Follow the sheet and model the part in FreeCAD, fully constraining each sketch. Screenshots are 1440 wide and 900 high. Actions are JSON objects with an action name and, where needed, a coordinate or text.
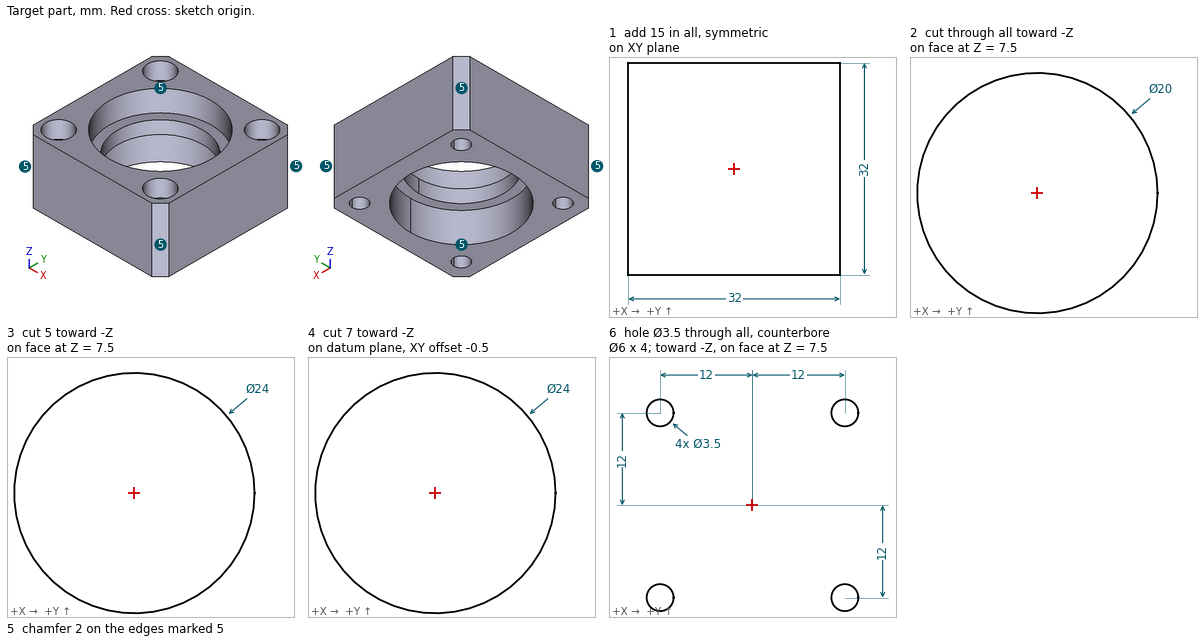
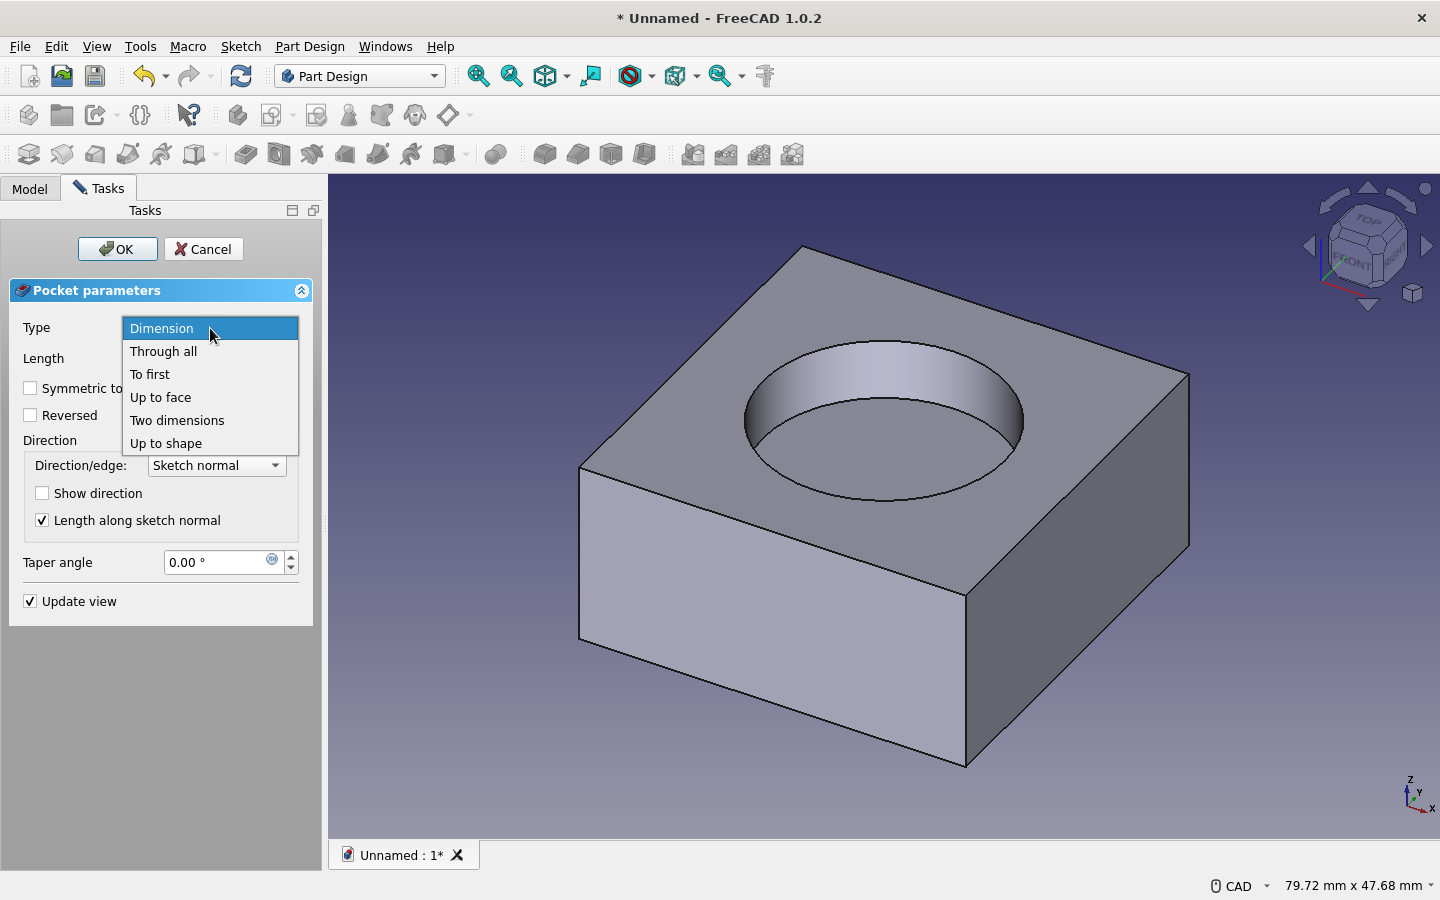
{"action": "left_click", "coordinate": [208, 352]}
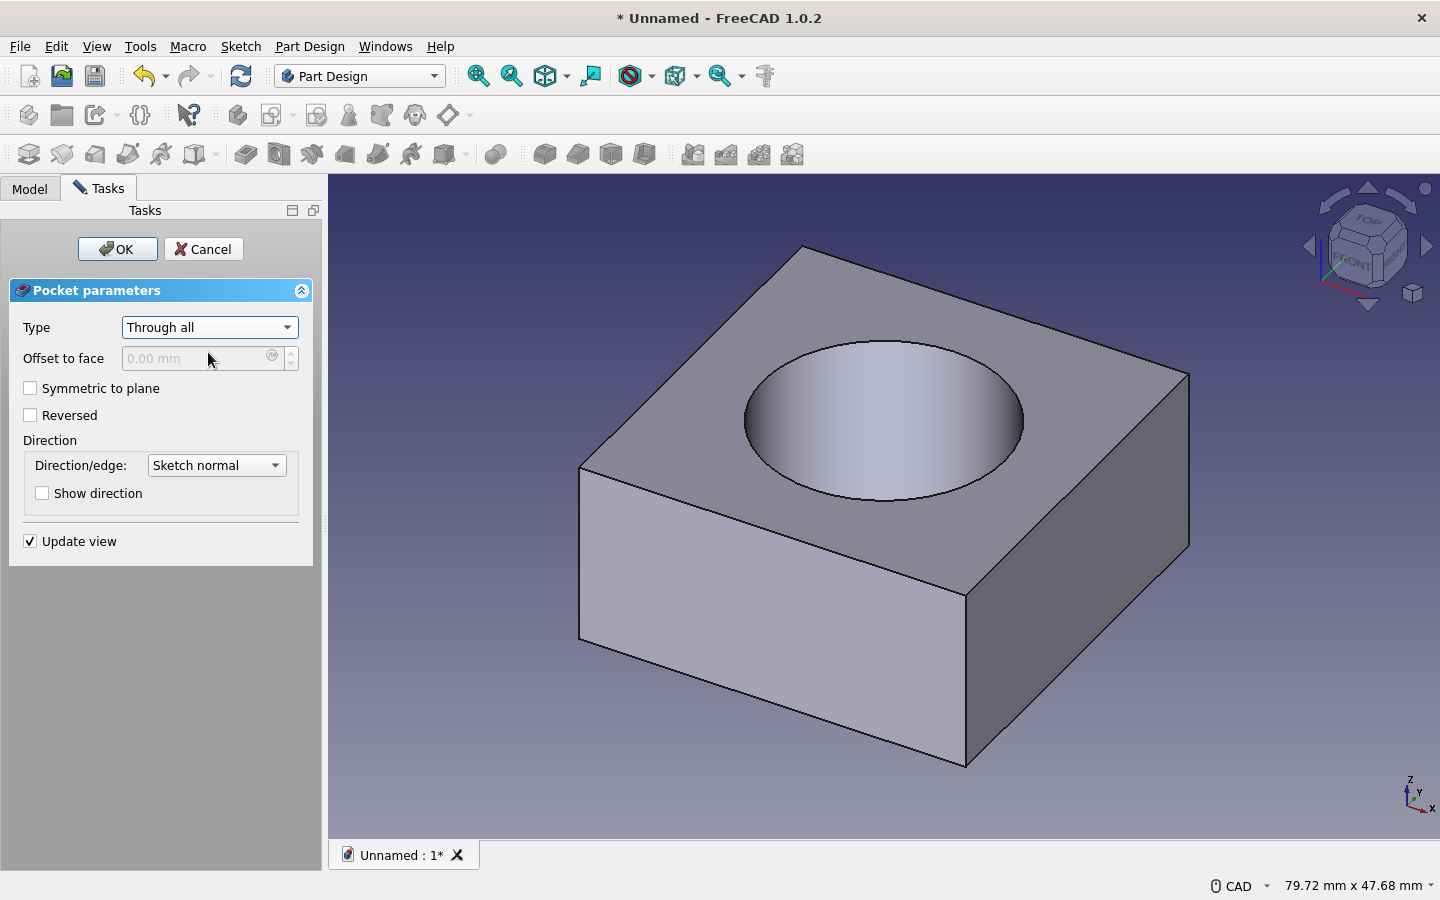
{"action": "left_click", "coordinate": [118, 249]}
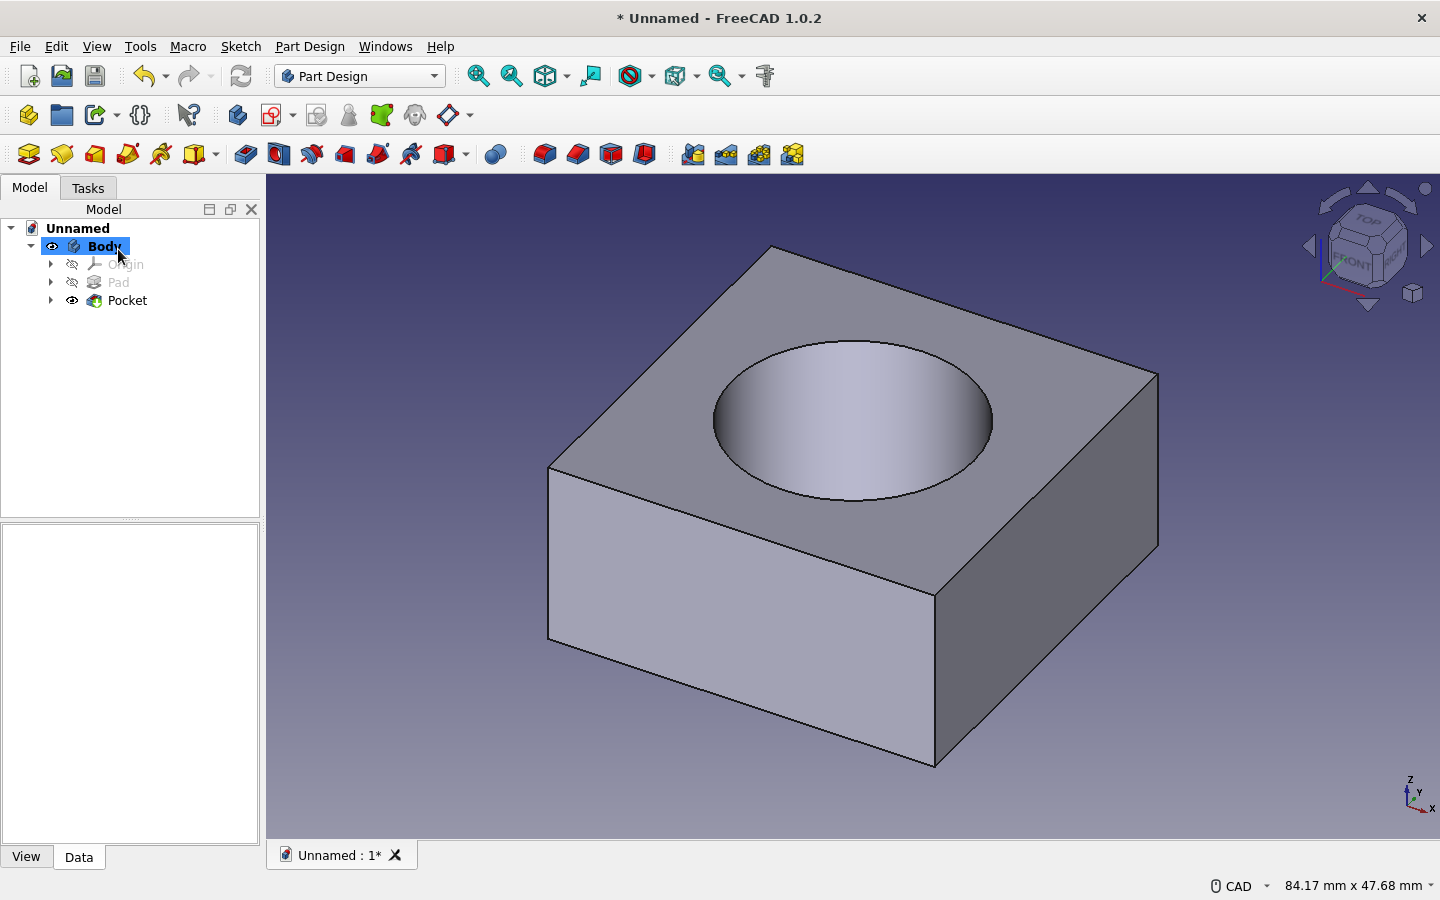
{"action": "left_click", "coordinate": [1027, 393]}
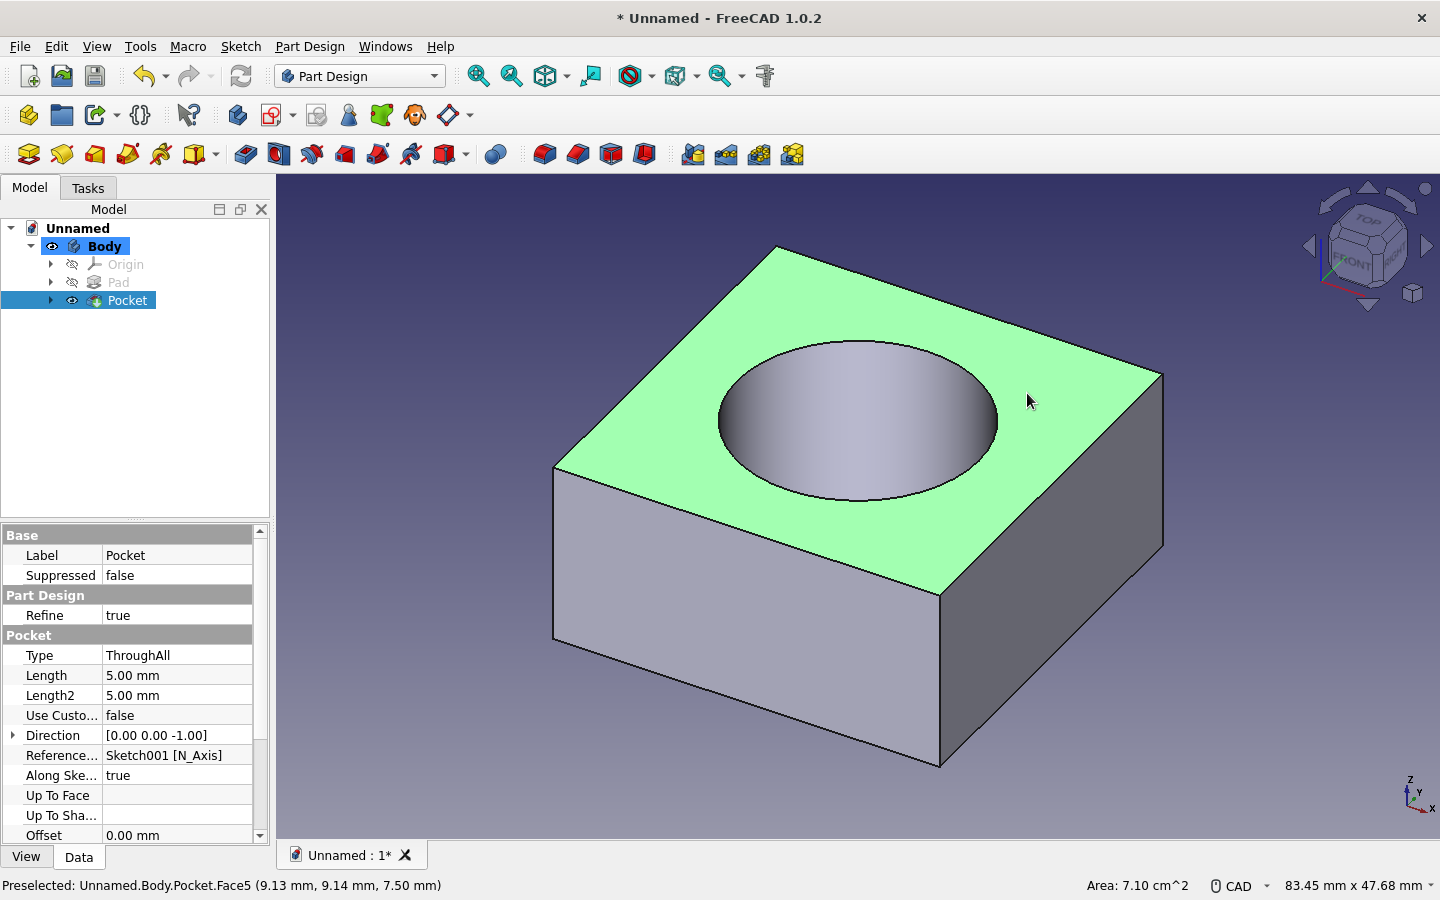
{"action": "left_click", "coordinate": [270, 116]}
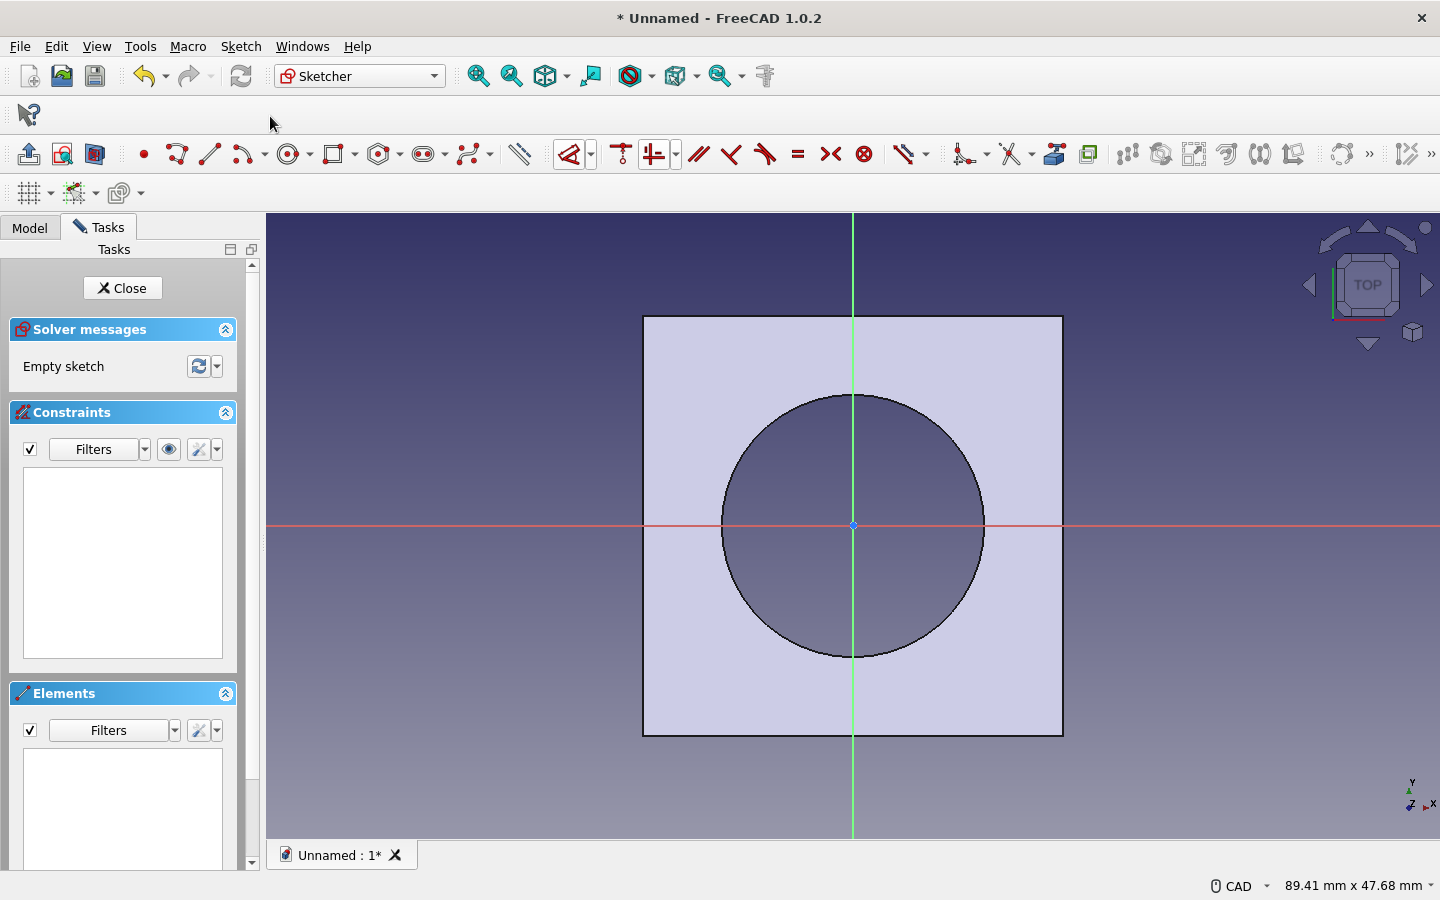
{"action": "left_click", "coordinate": [288, 154]}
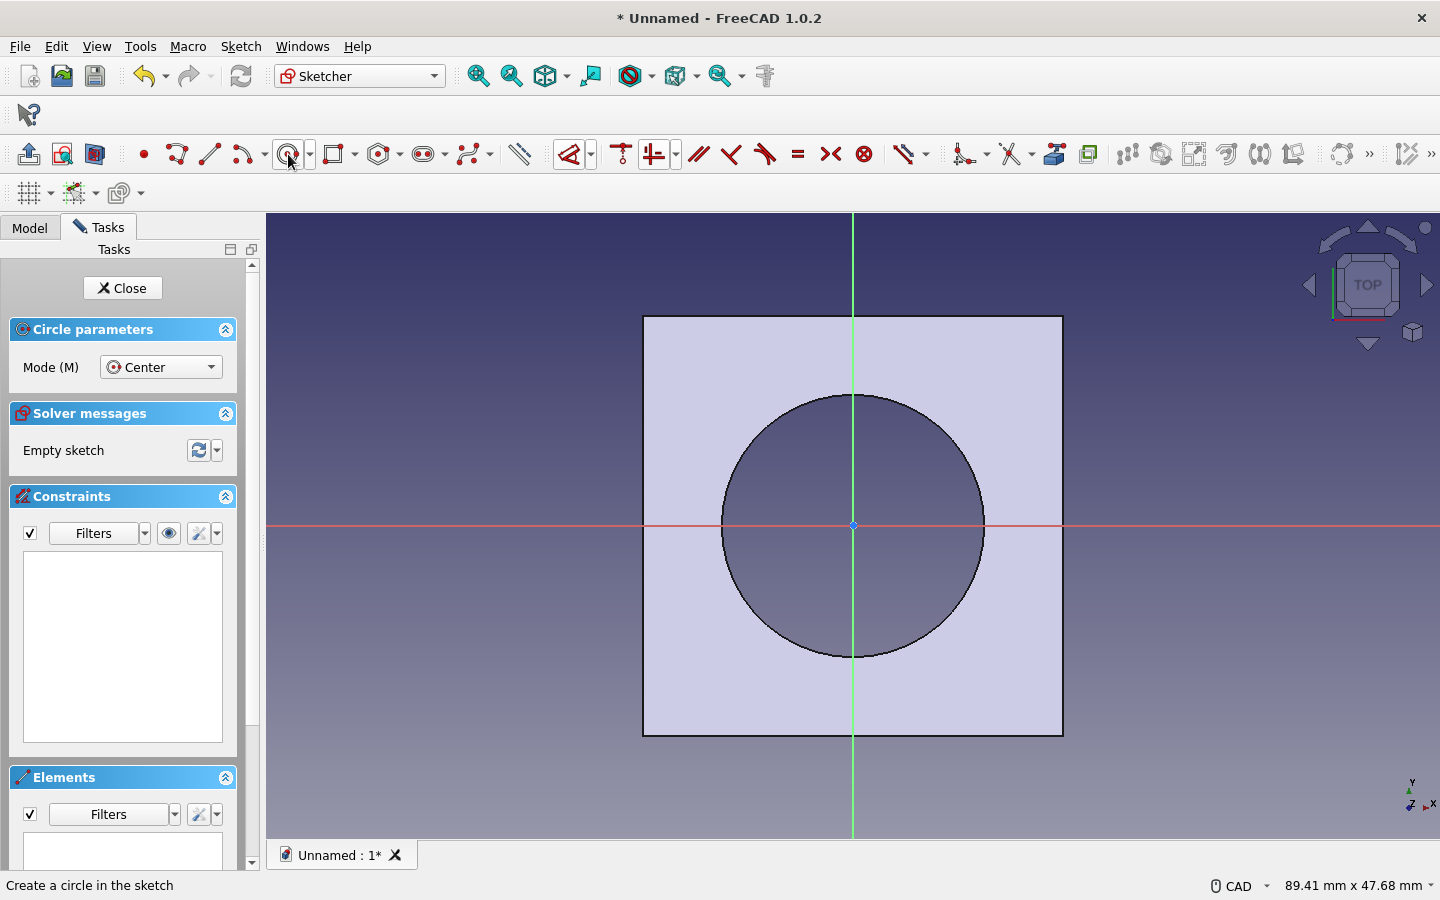
{"action": "left_click", "coordinate": [853, 526]}
{"action": "left_click", "coordinate": [964, 415]}
{"action": "key", "text": "Escape"}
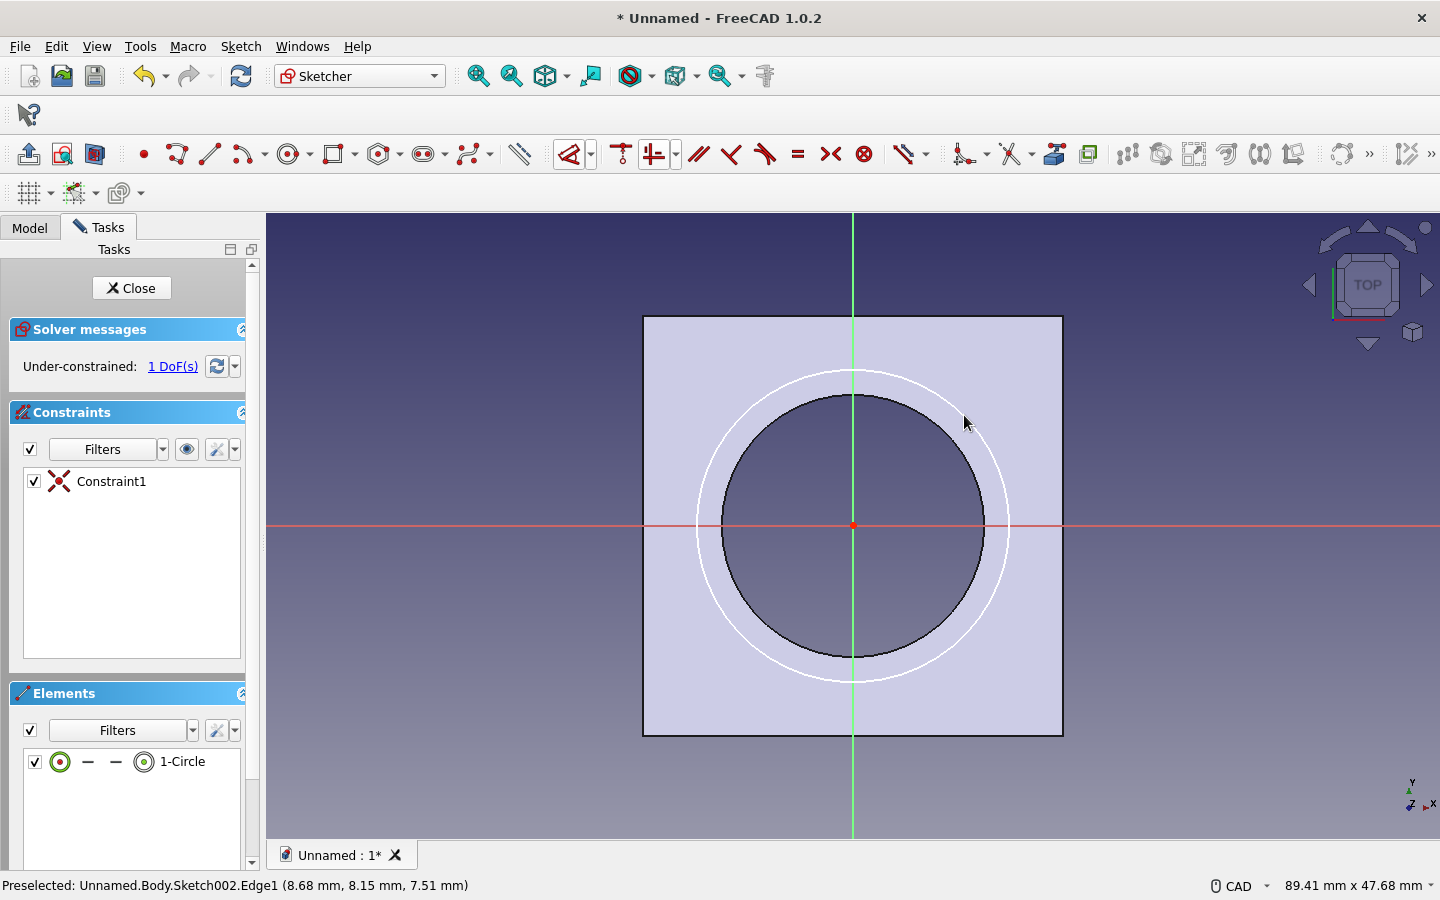
{"action": "left_click", "coordinate": [963, 415]}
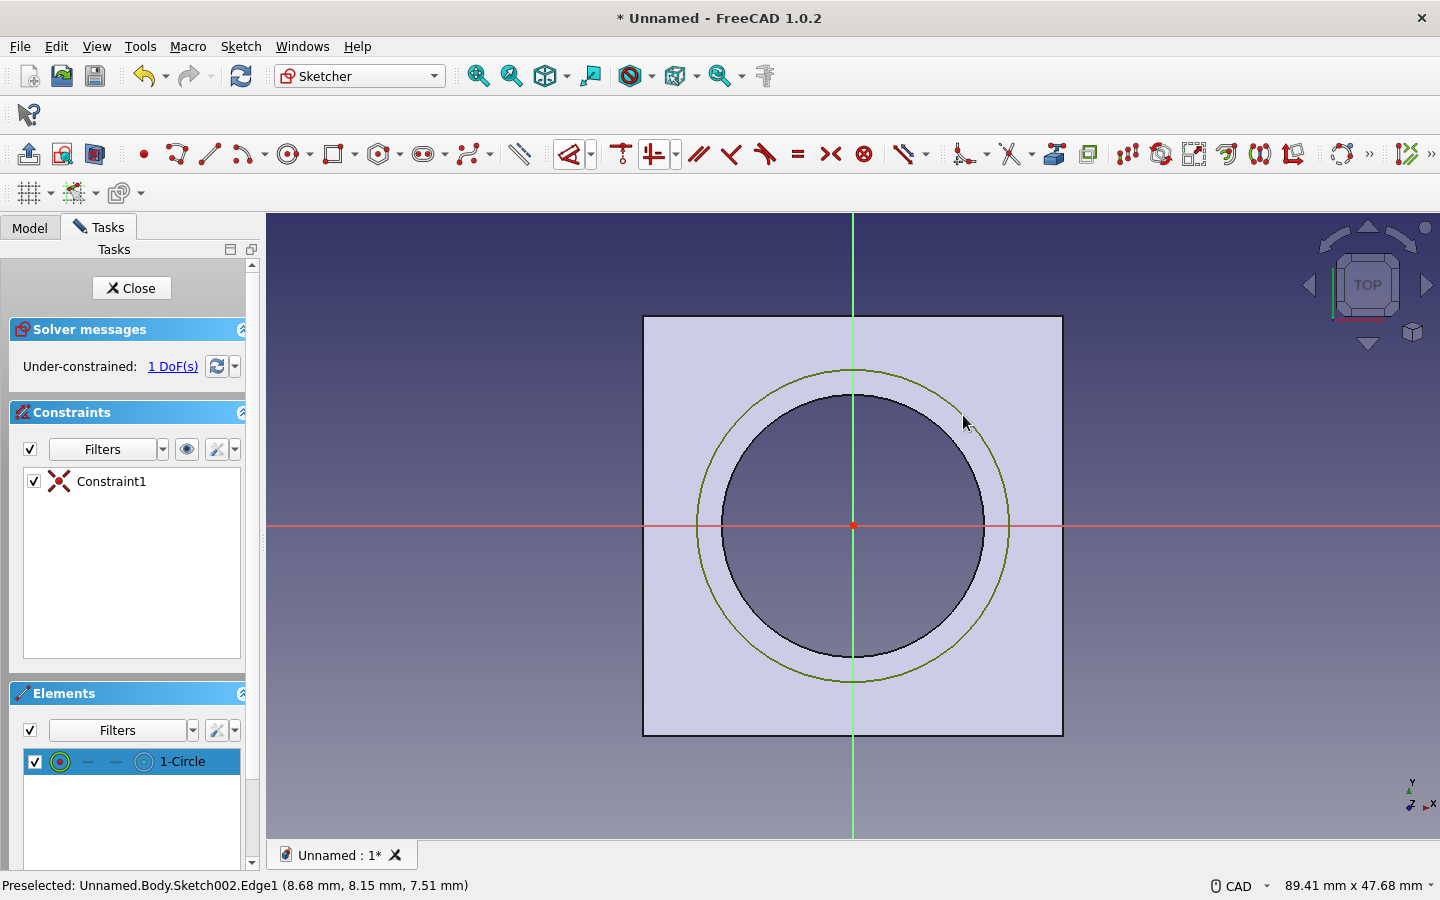
{"action": "key", "text": "k o"}